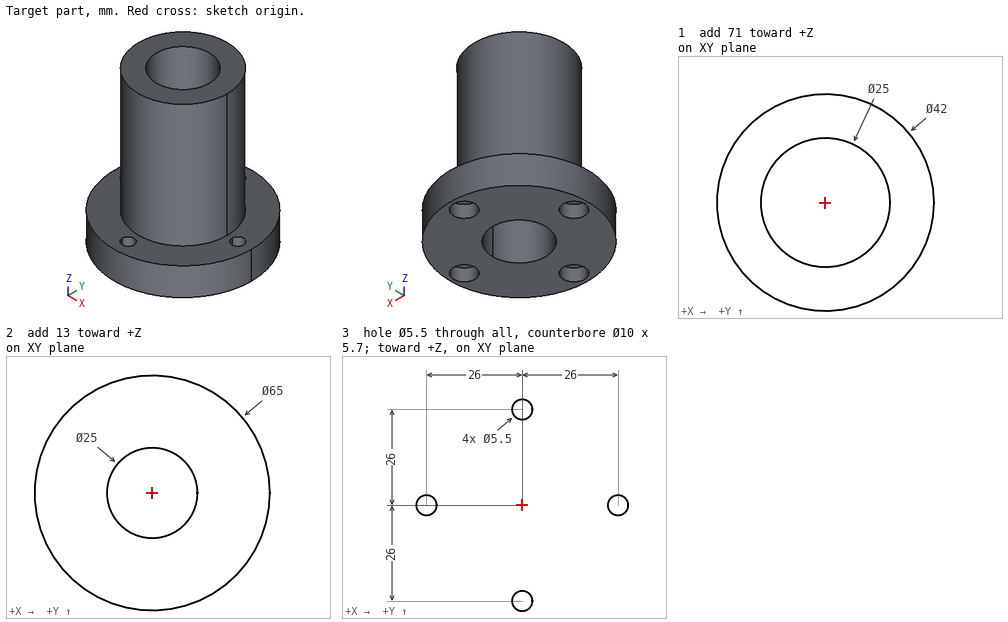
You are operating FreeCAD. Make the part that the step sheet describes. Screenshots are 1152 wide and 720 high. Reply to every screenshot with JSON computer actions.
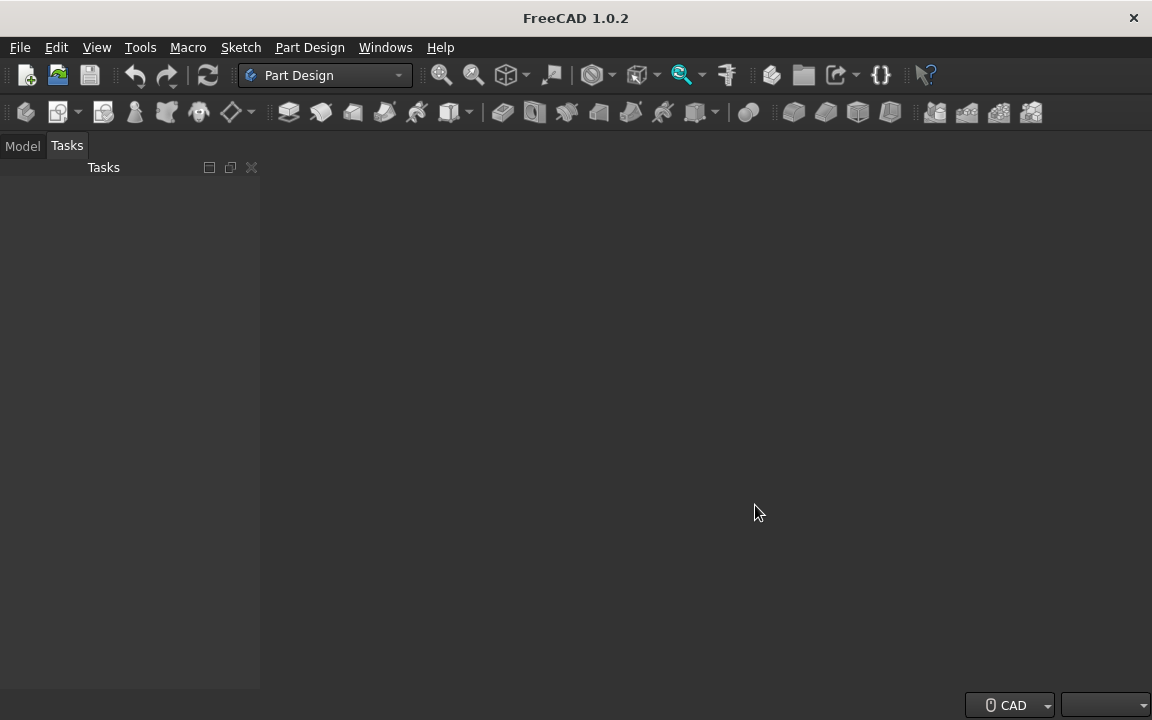
{"action": "left_click", "coordinate": [26, 76]}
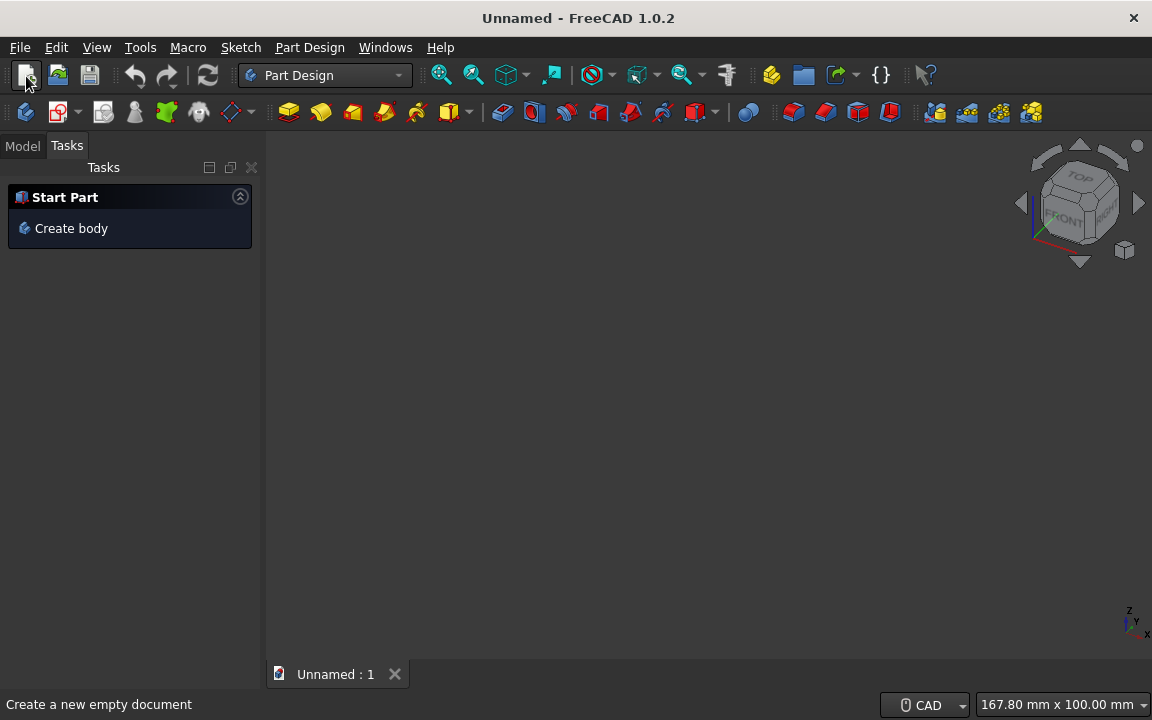
{"action": "left_click", "coordinate": [58, 112]}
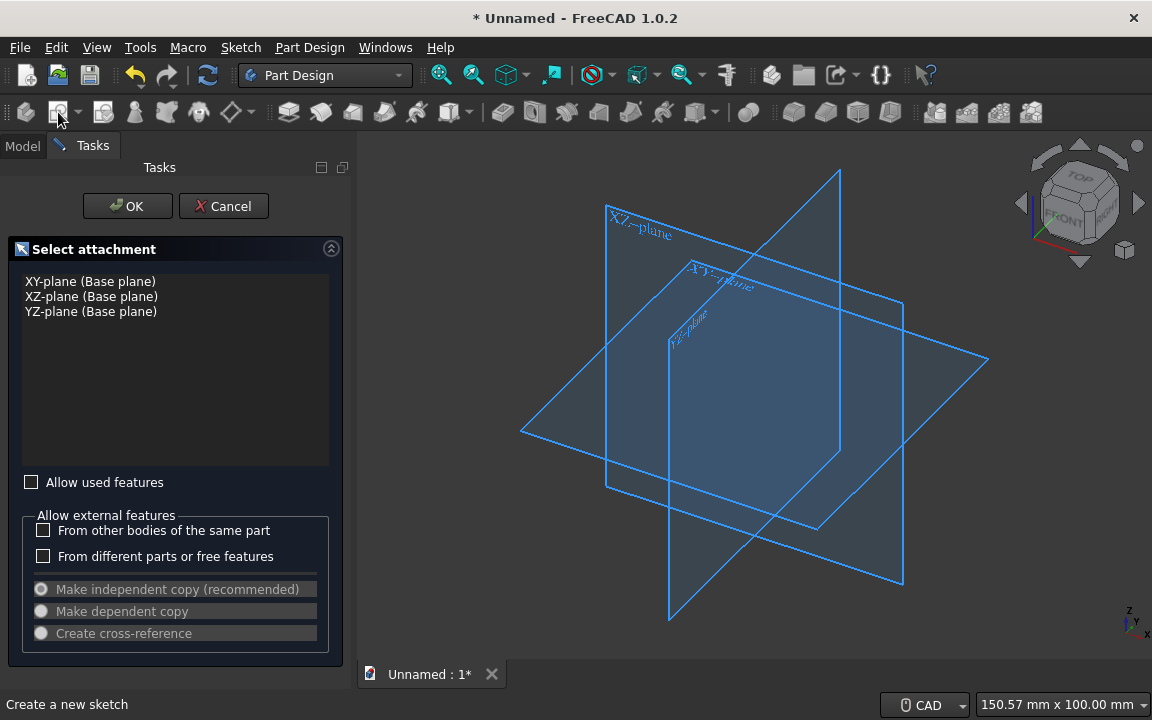
{"action": "left_click", "coordinate": [82, 282]}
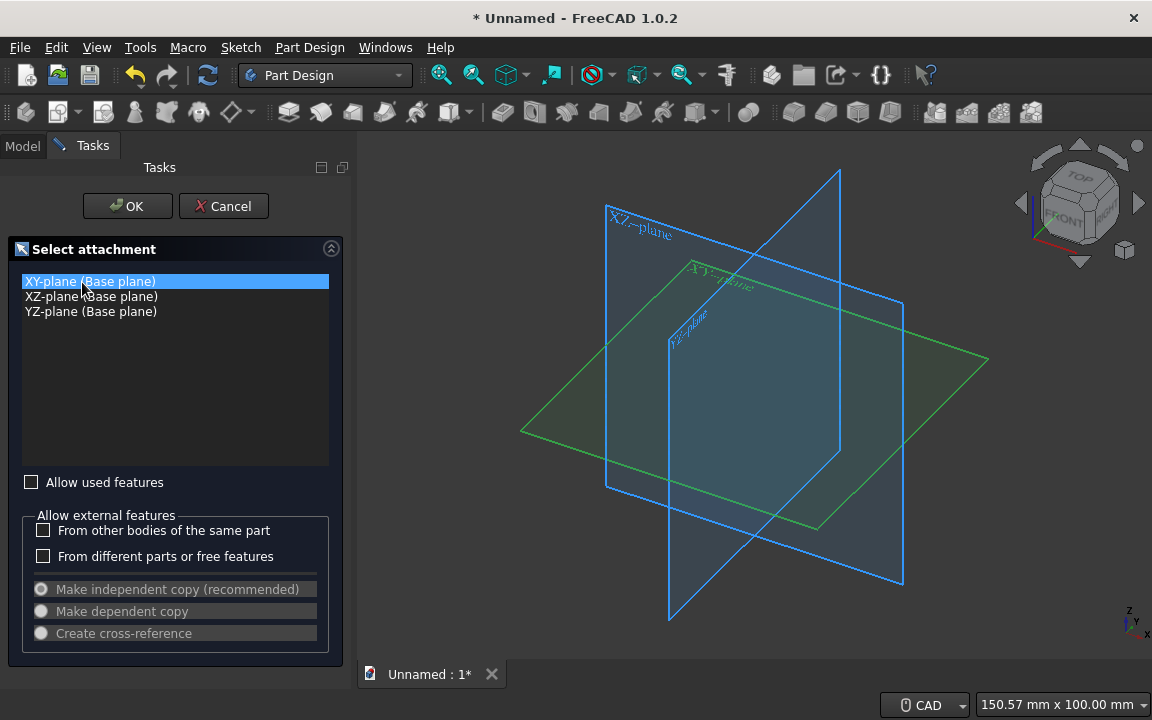
{"action": "left_click", "coordinate": [128, 206]}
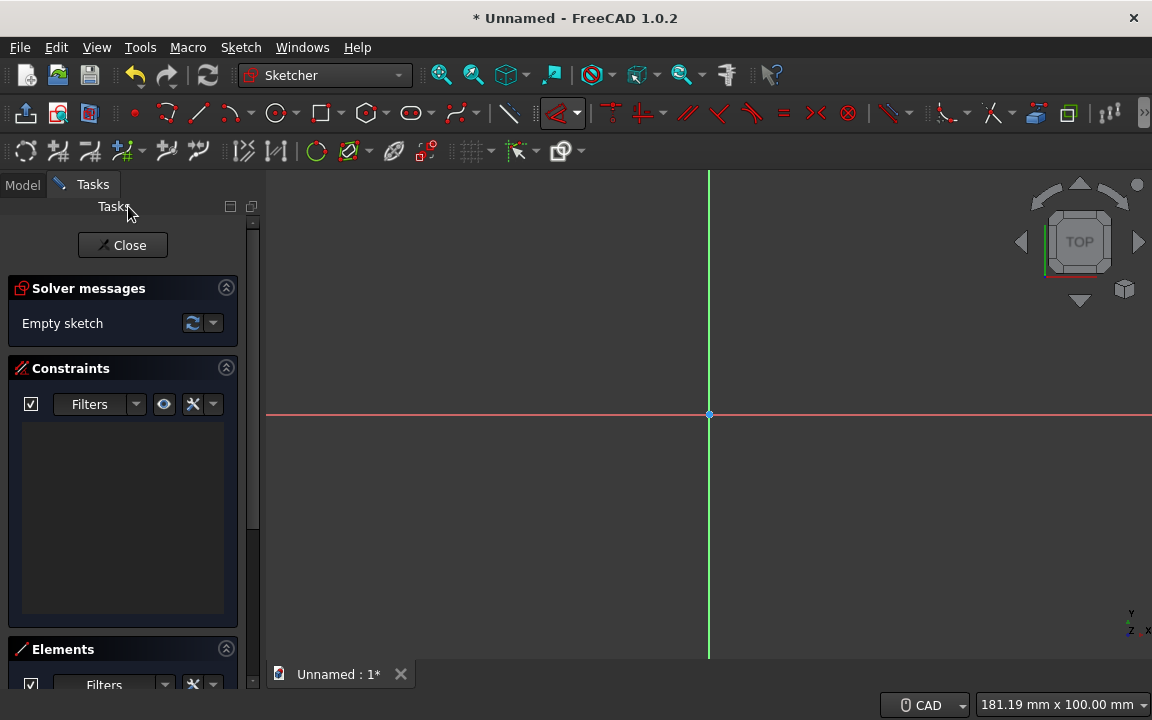
{"action": "scroll", "coordinate": [848, 414], "scroll_direction": "up", "scroll_amount": 2}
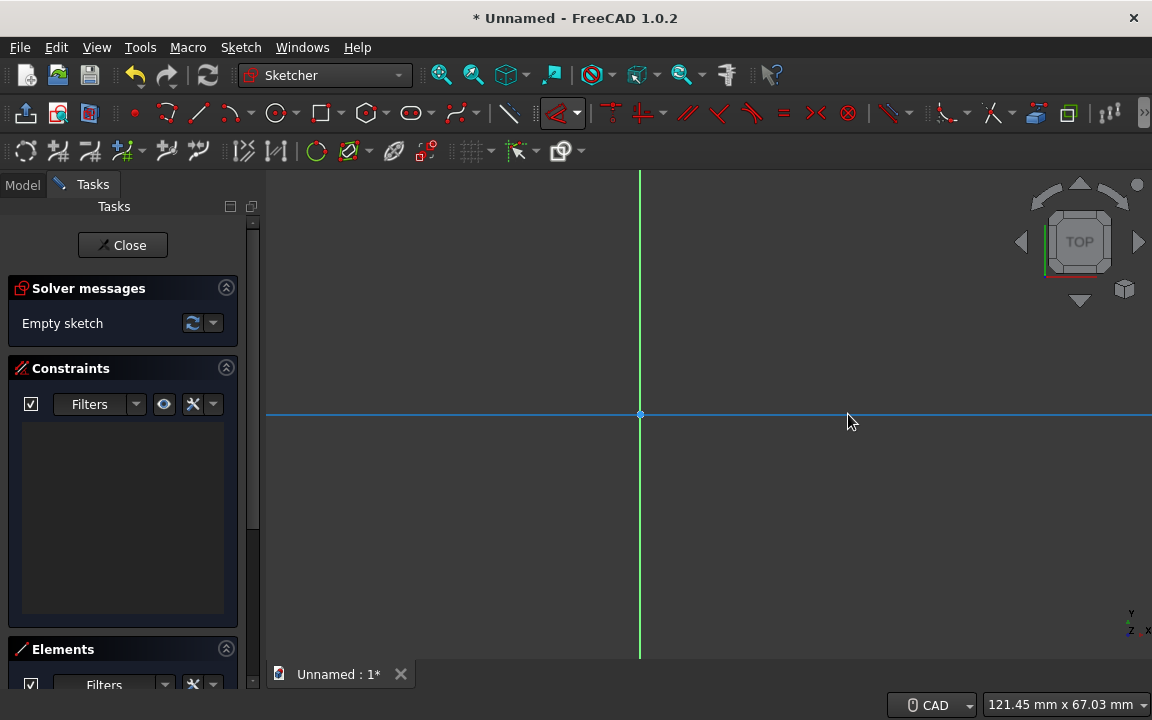
{"action": "left_click", "coordinate": [276, 114]}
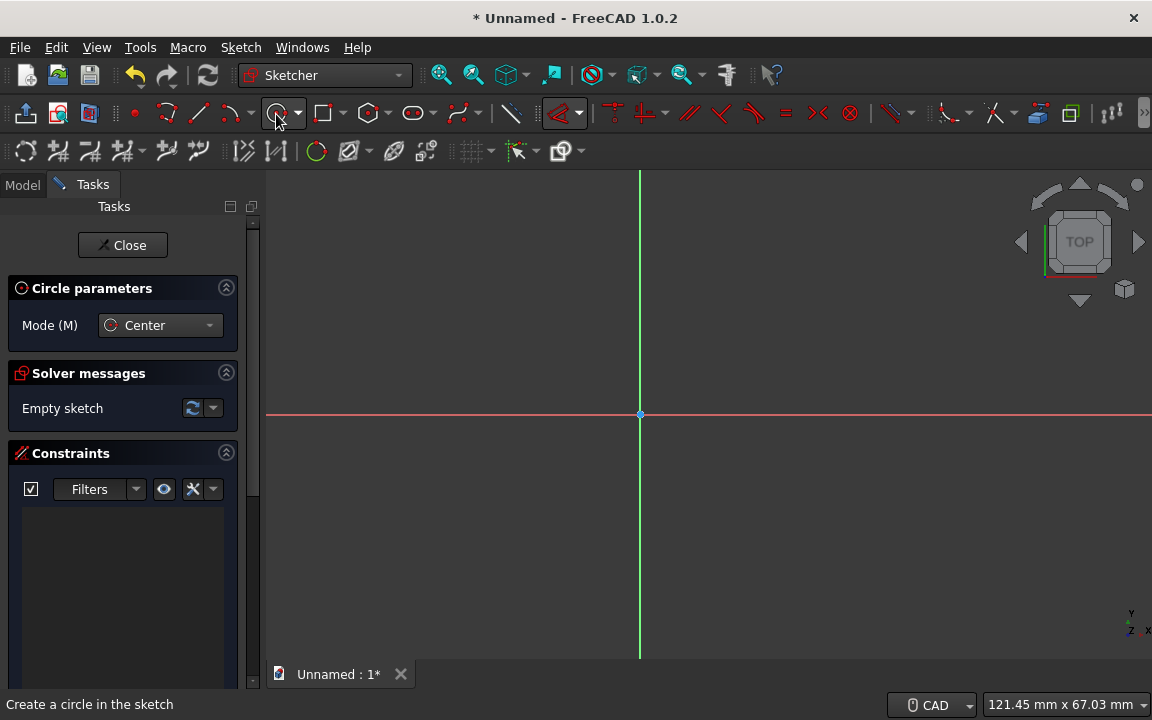
{"action": "left_click", "coordinate": [640, 414]}
{"action": "mouse_move", "coordinate": [749, 306]}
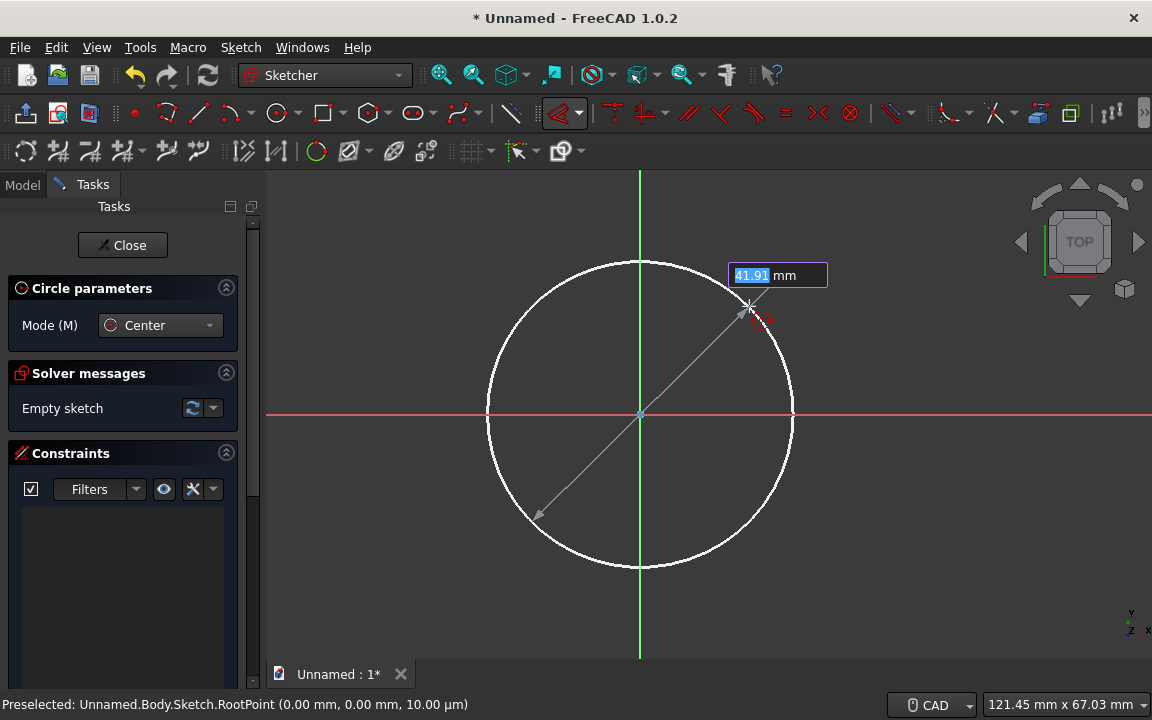
{"action": "type", "text": "42"}
{"action": "key", "text": "Return"}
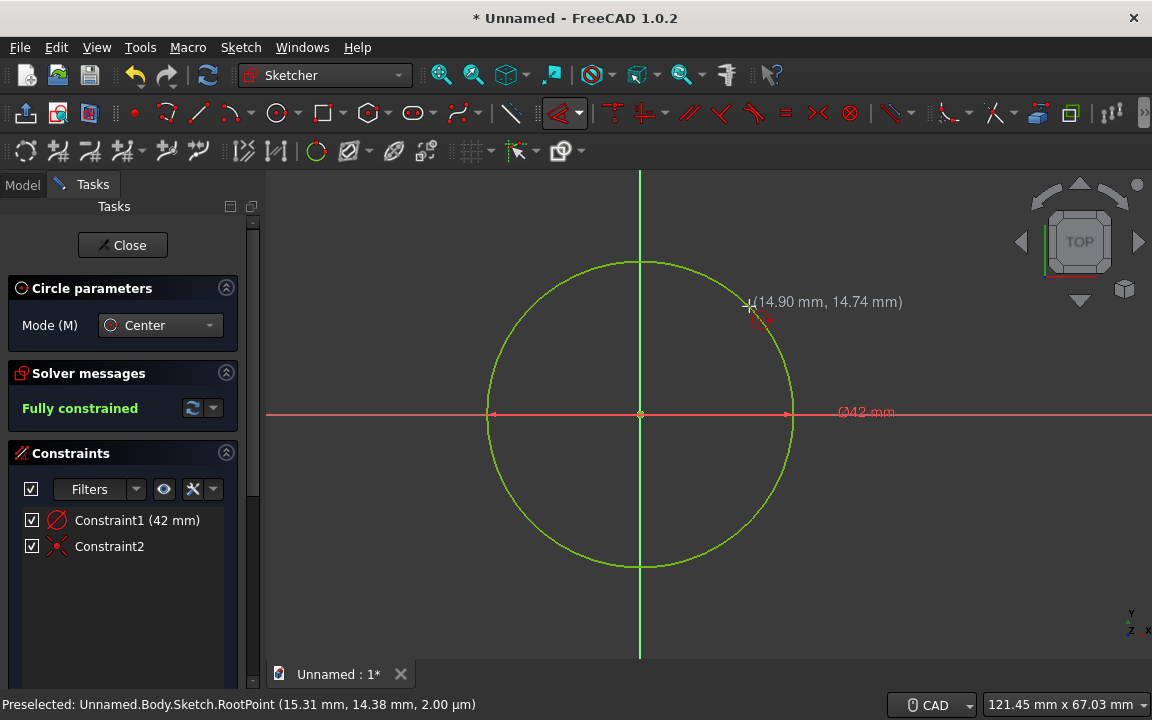
{"action": "left_click", "coordinate": [640, 414]}
{"action": "mouse_move", "coordinate": [705, 350]}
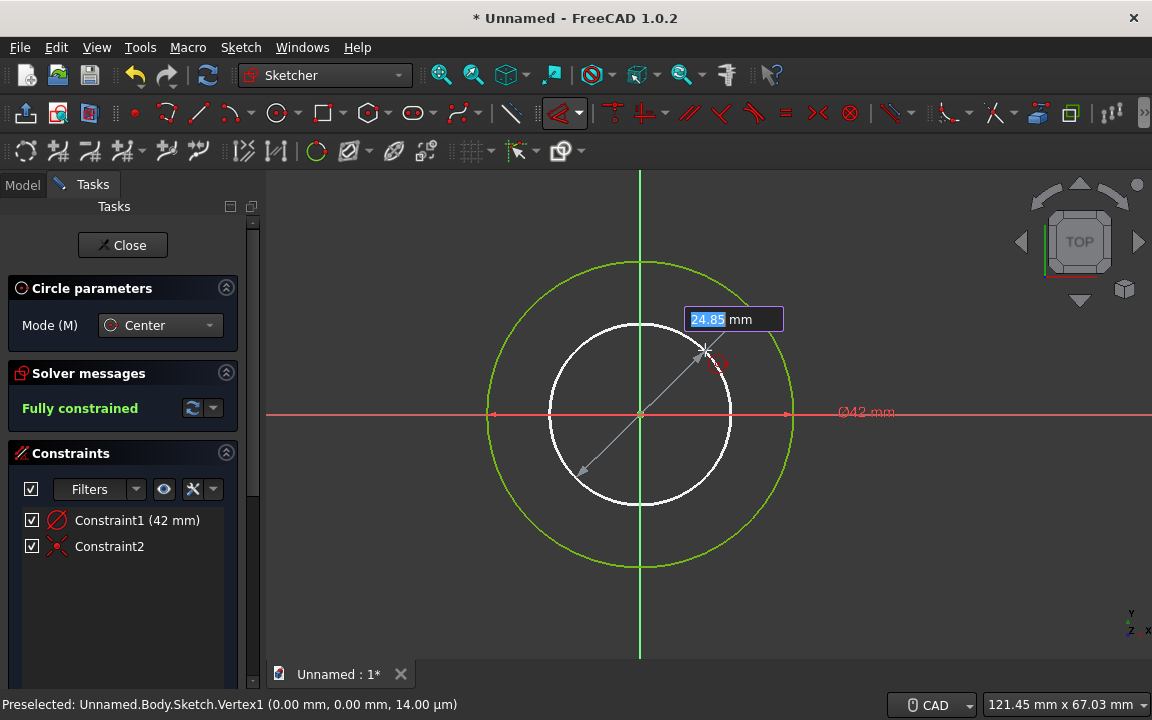
{"action": "type", "text": "25"}
{"action": "key", "text": "Return"}
{"action": "key", "text": "Escape"}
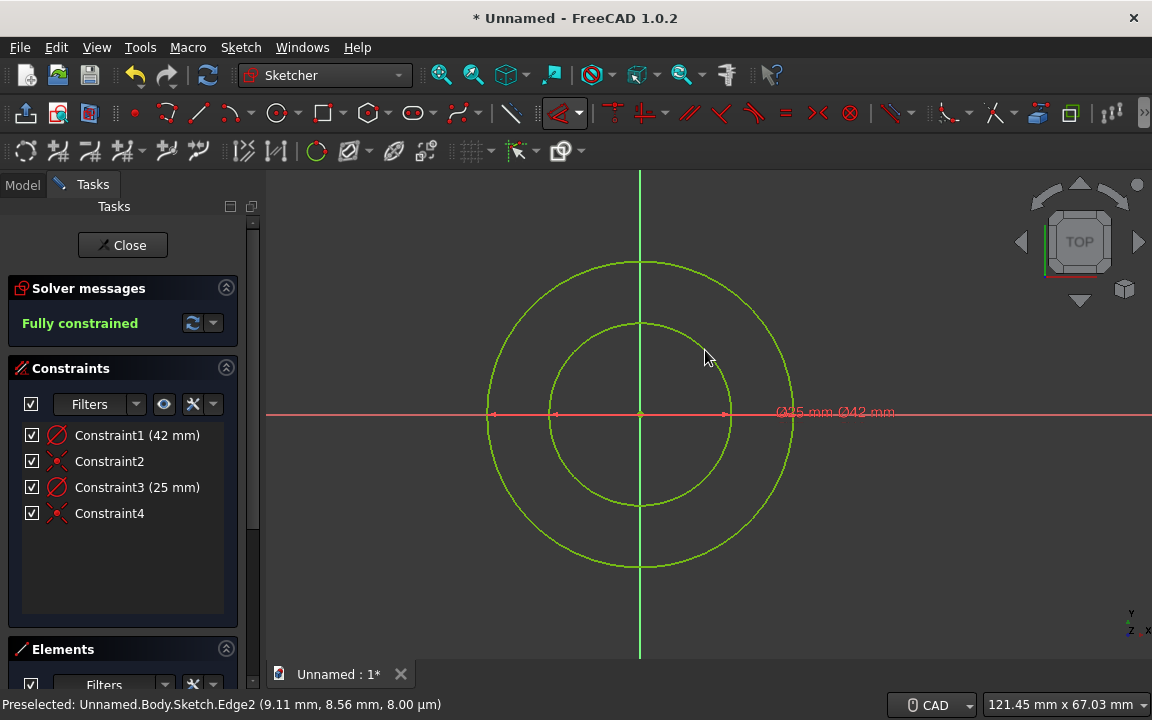
{"action": "left_click", "coordinate": [123, 245]}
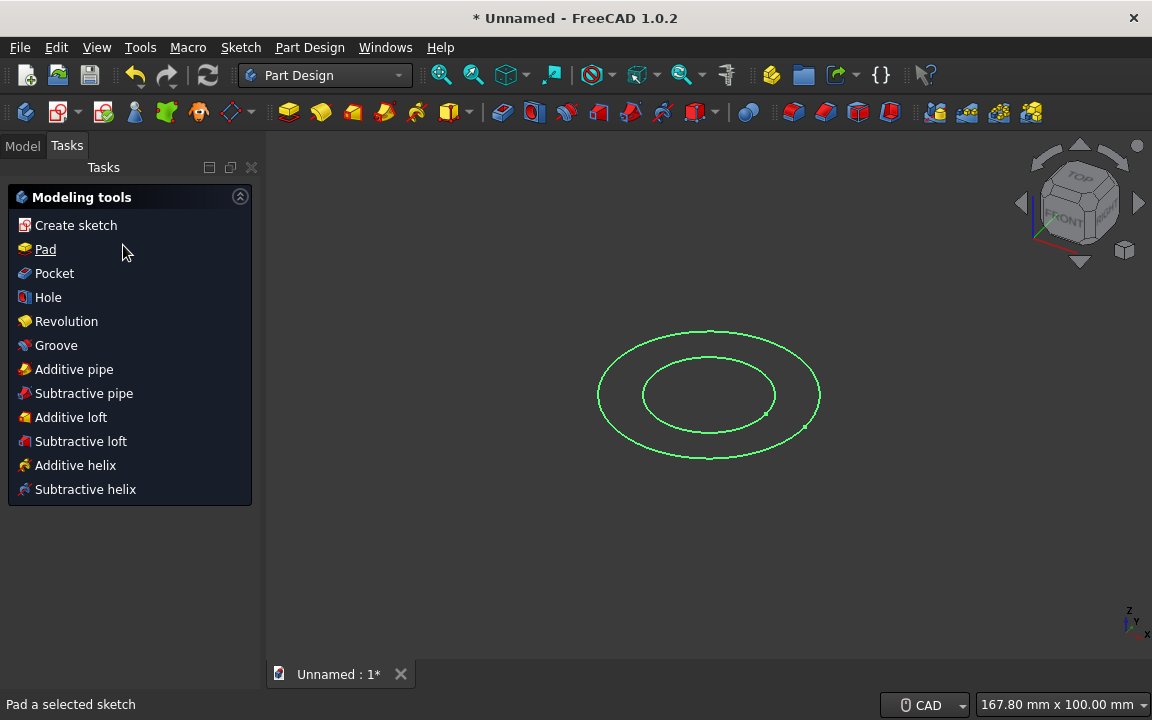
{"action": "left_click", "coordinate": [290, 112]}